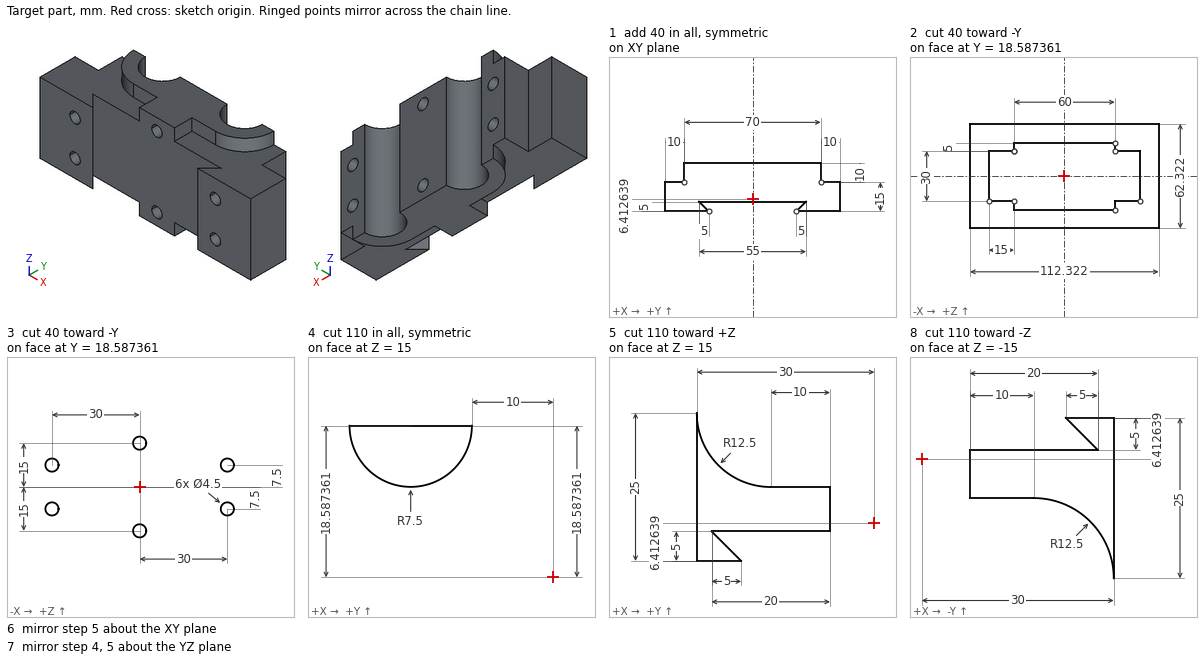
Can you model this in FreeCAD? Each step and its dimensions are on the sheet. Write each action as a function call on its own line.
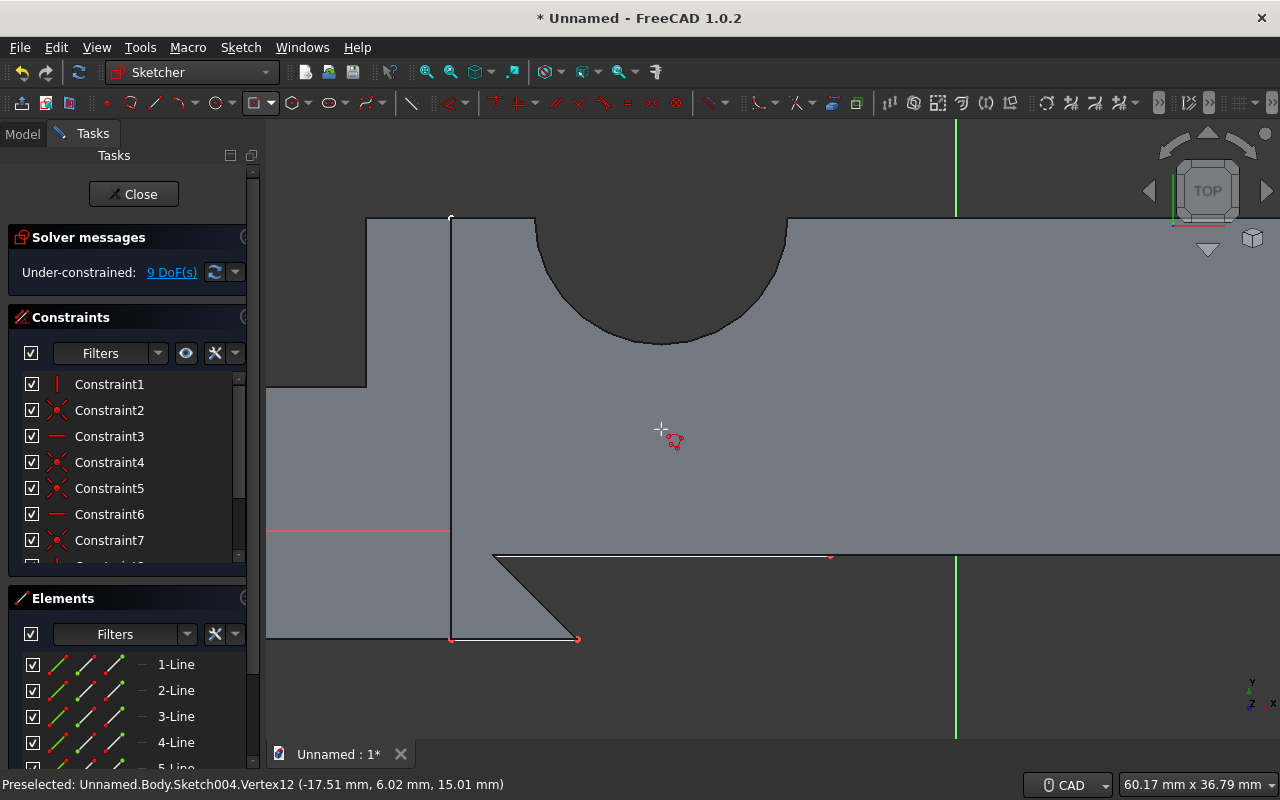
click(180, 104)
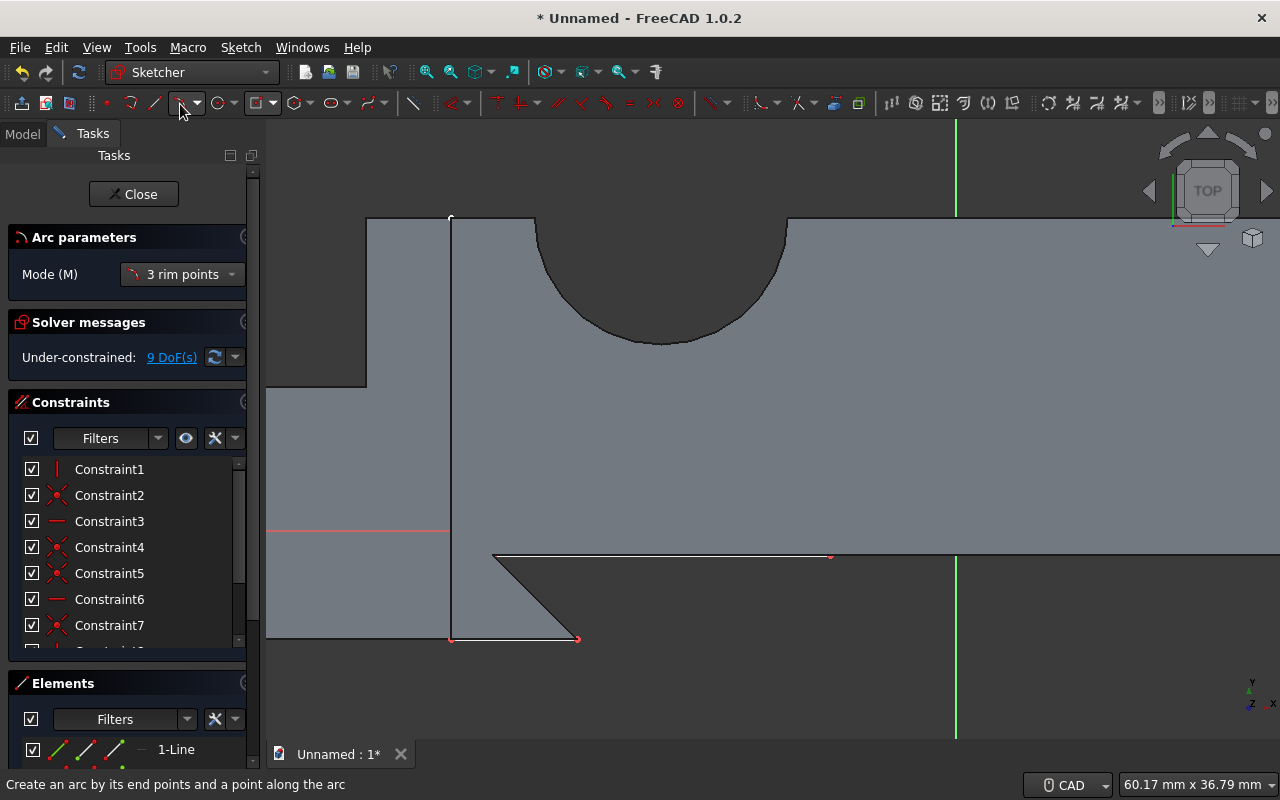
click(661, 430)
click(451, 219)
click(512, 367)
key(Escape)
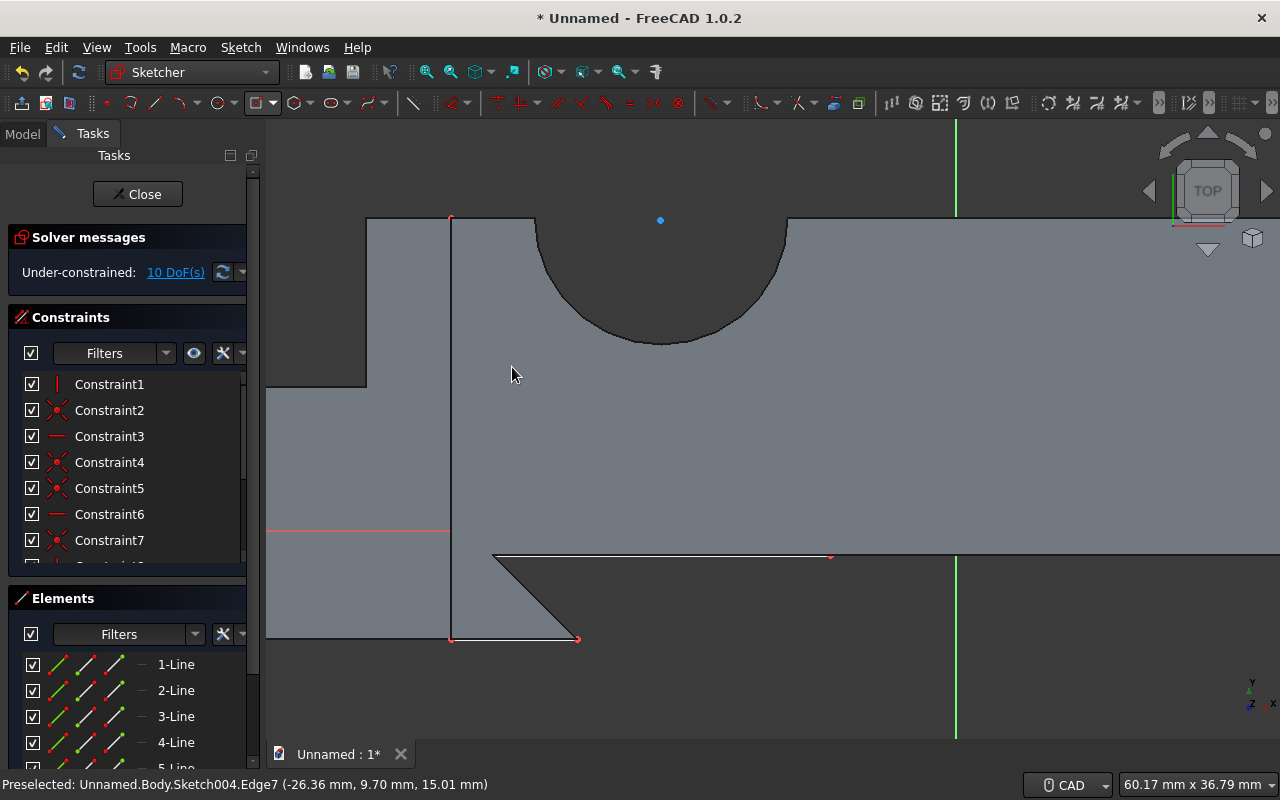
click(451, 345)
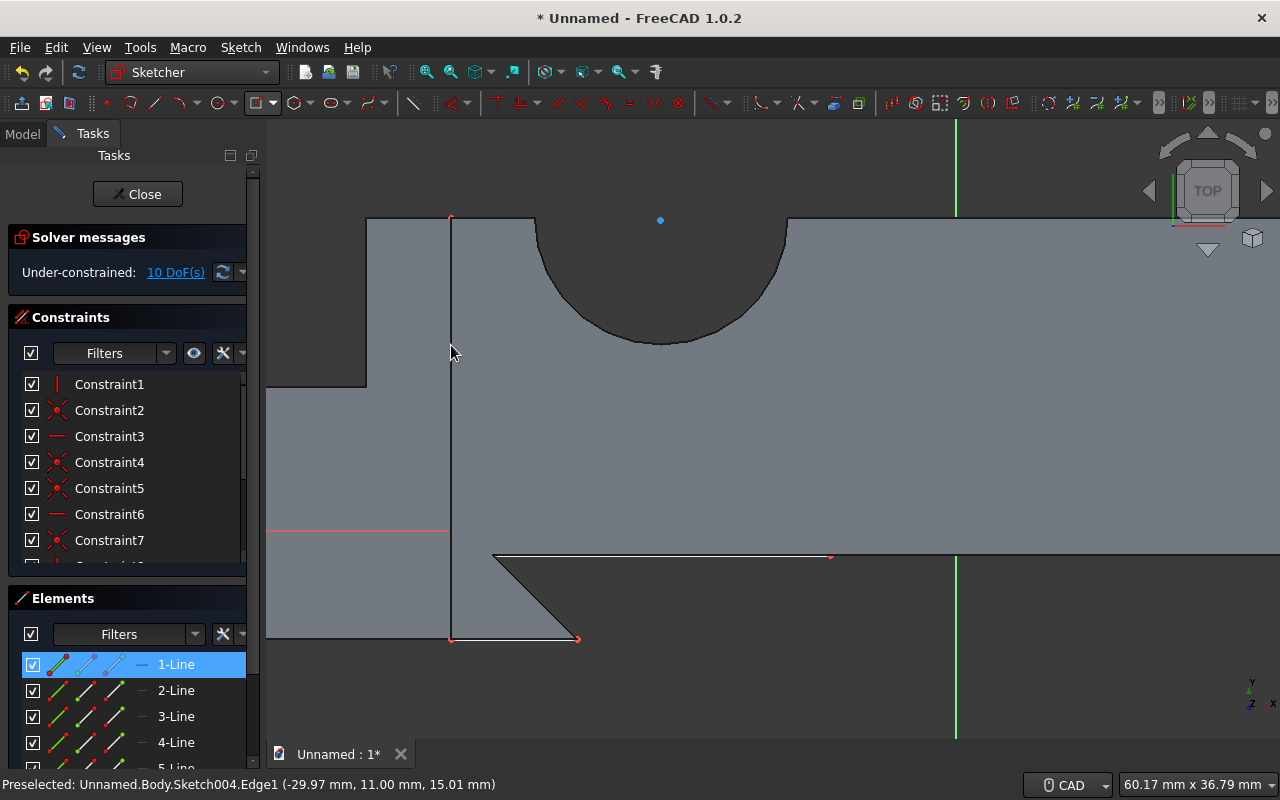
click(474, 315)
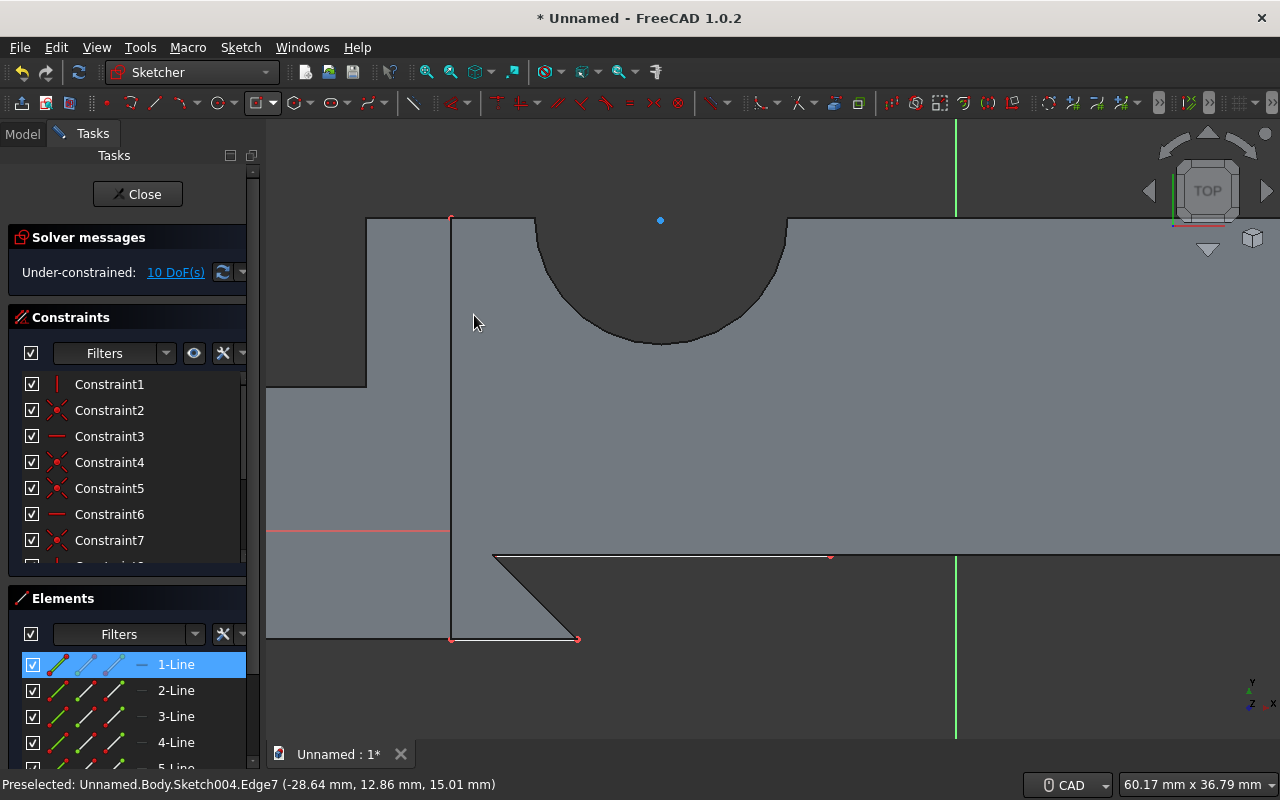
key(t)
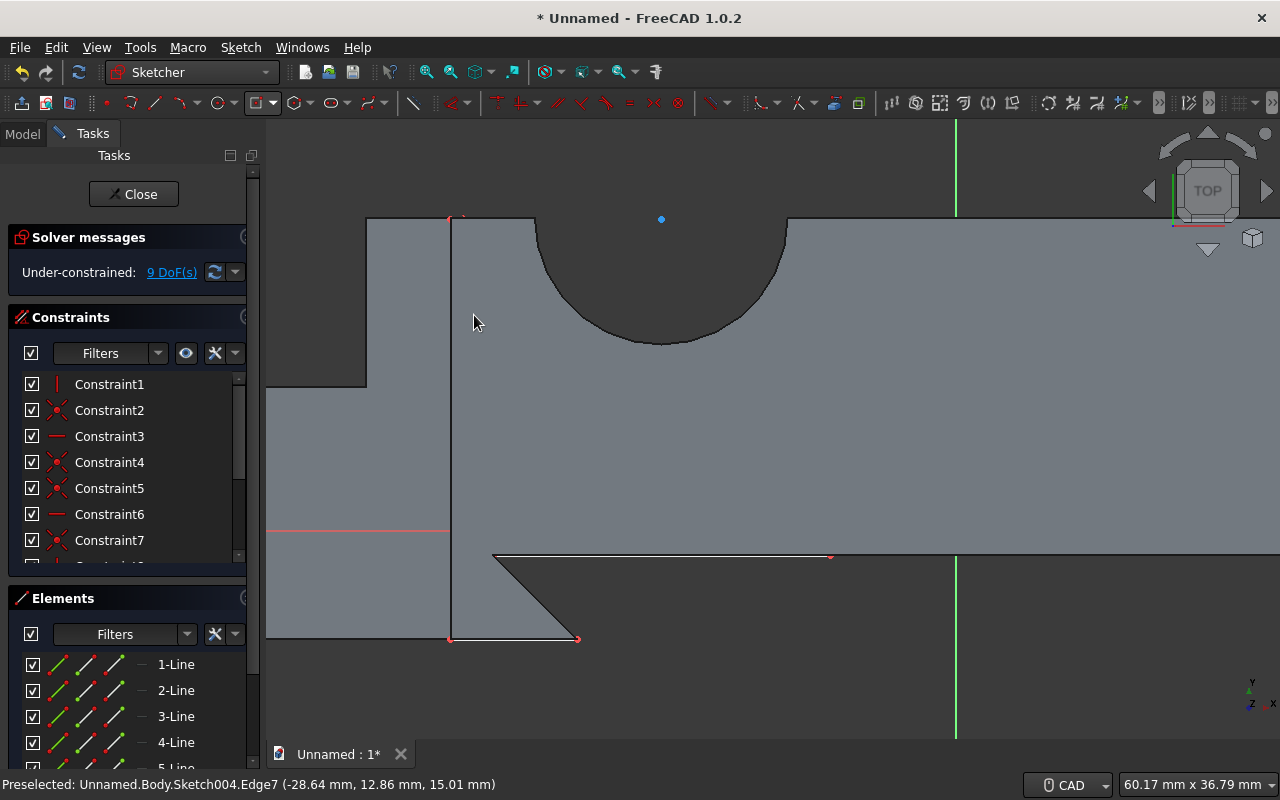
click(779, 430)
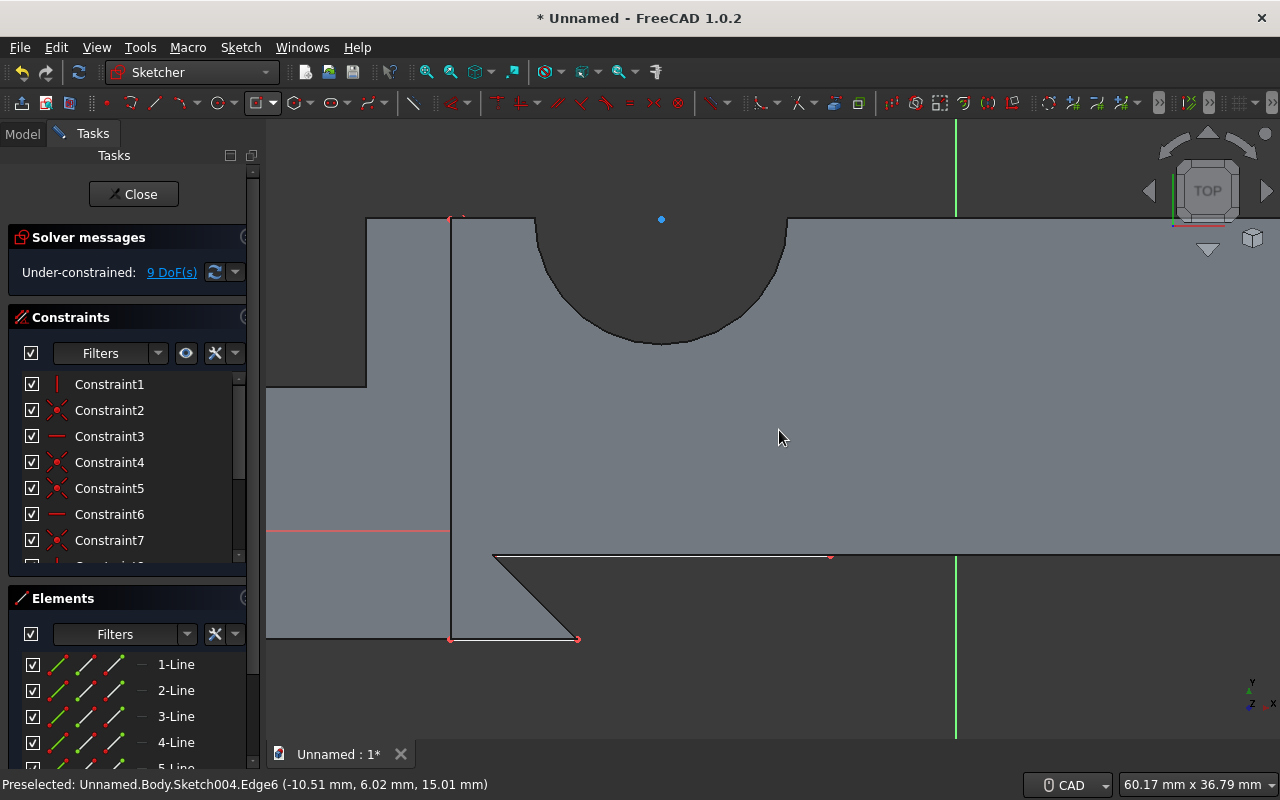
click(474, 315)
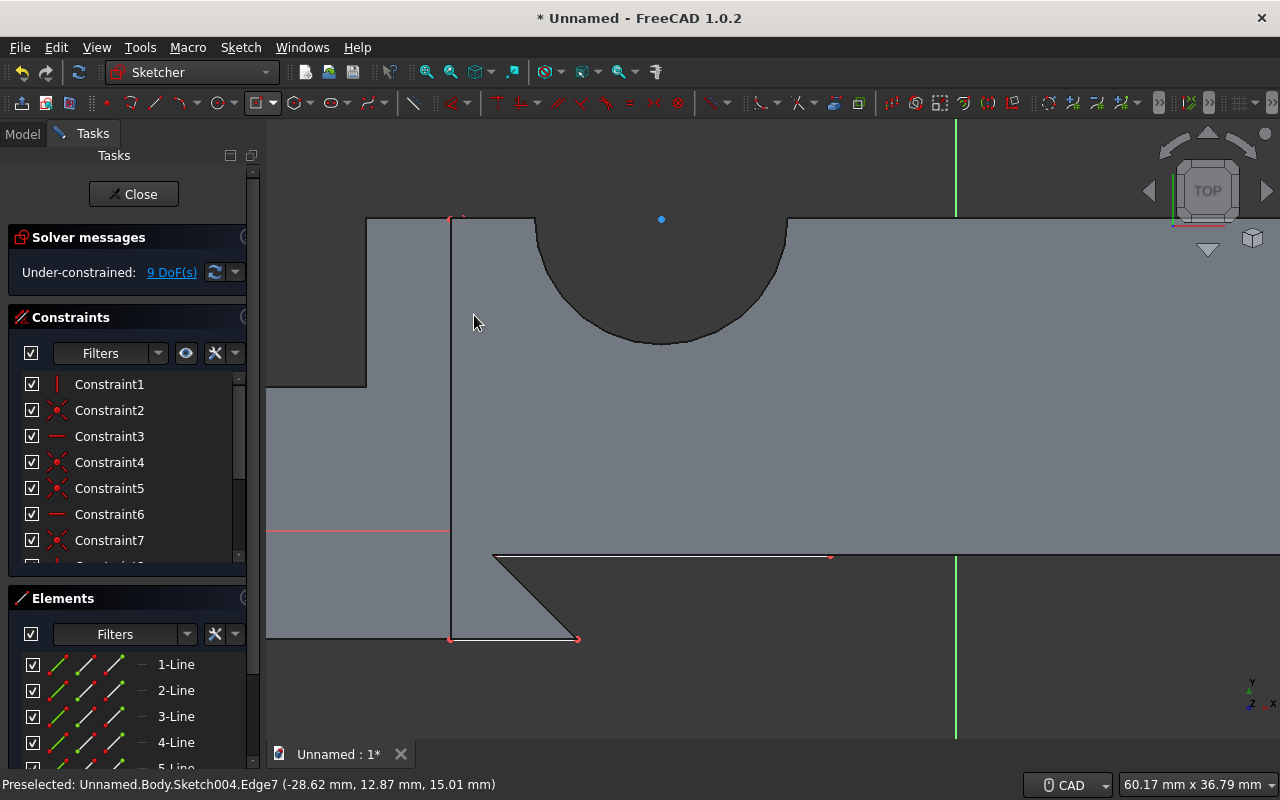
key(t)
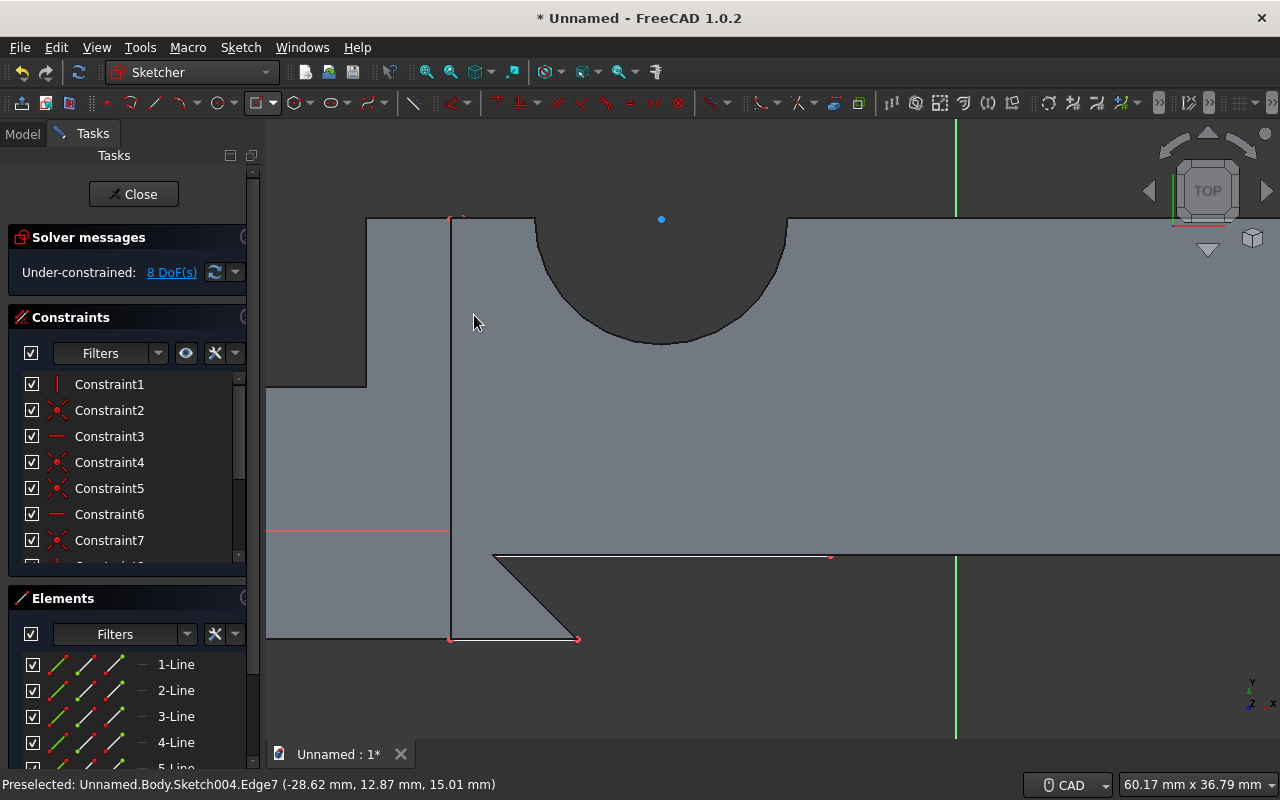
key(d)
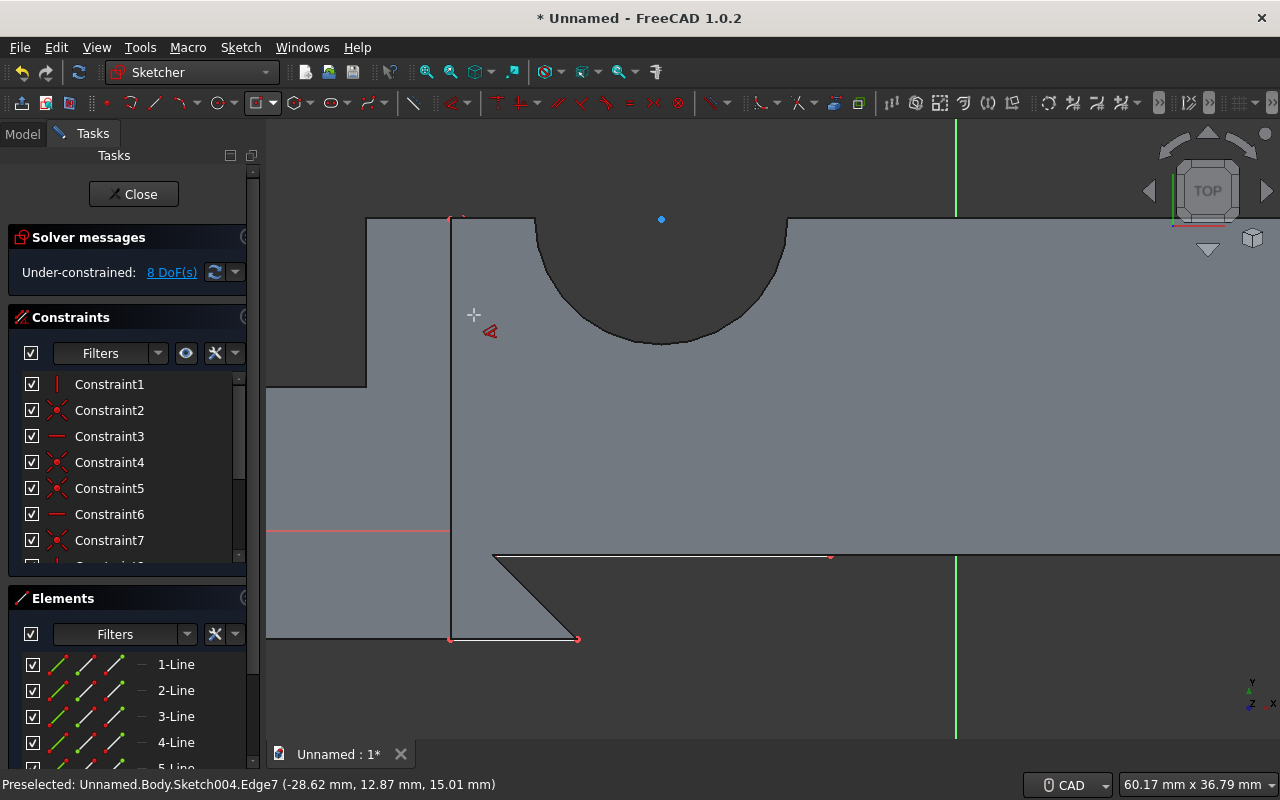
click(474, 315)
click(419, 212)